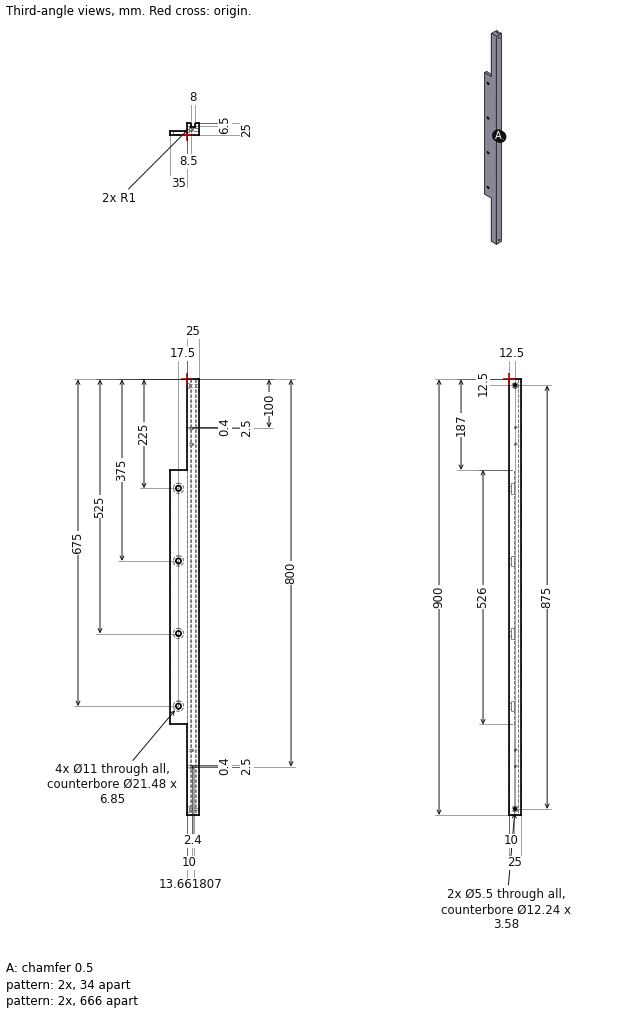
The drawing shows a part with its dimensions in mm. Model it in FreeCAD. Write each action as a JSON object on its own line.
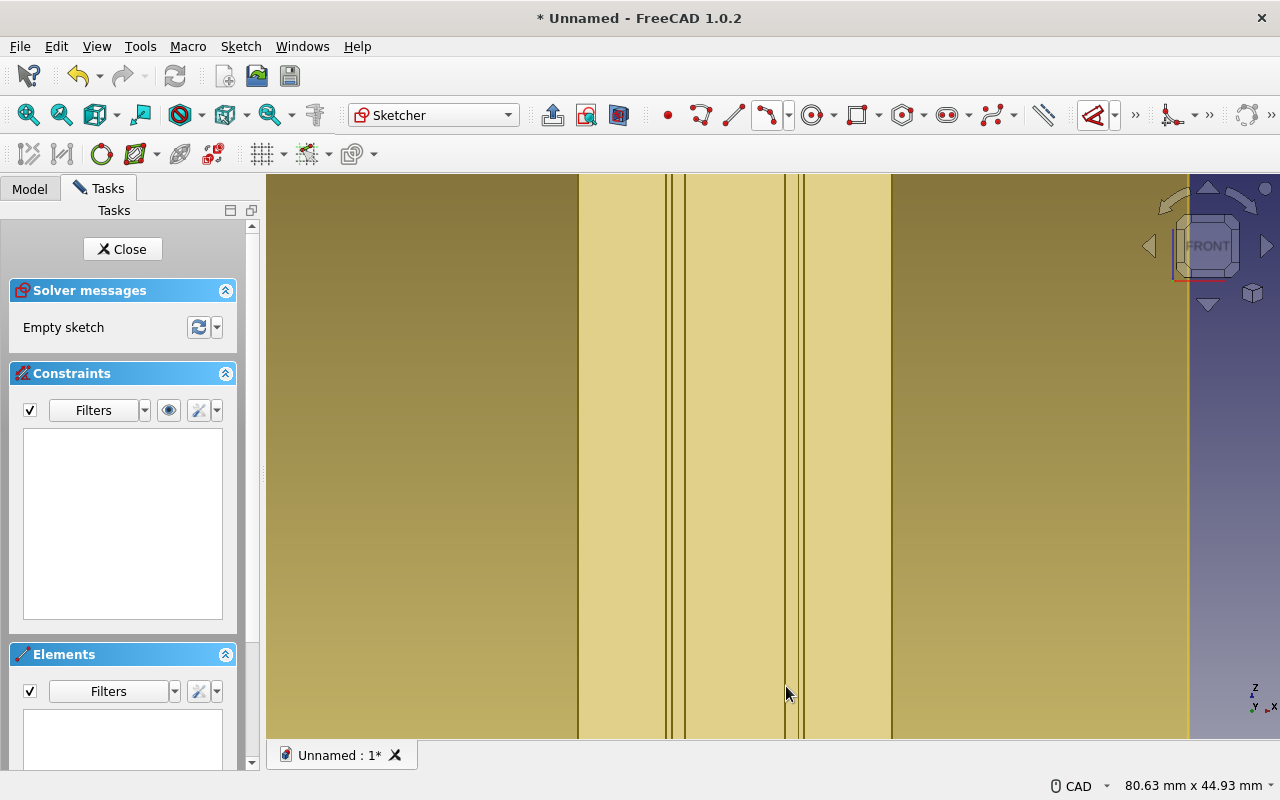
{"action": "scroll", "coordinate": [693, 436], "scroll_direction": "up", "scroll_amount": 4}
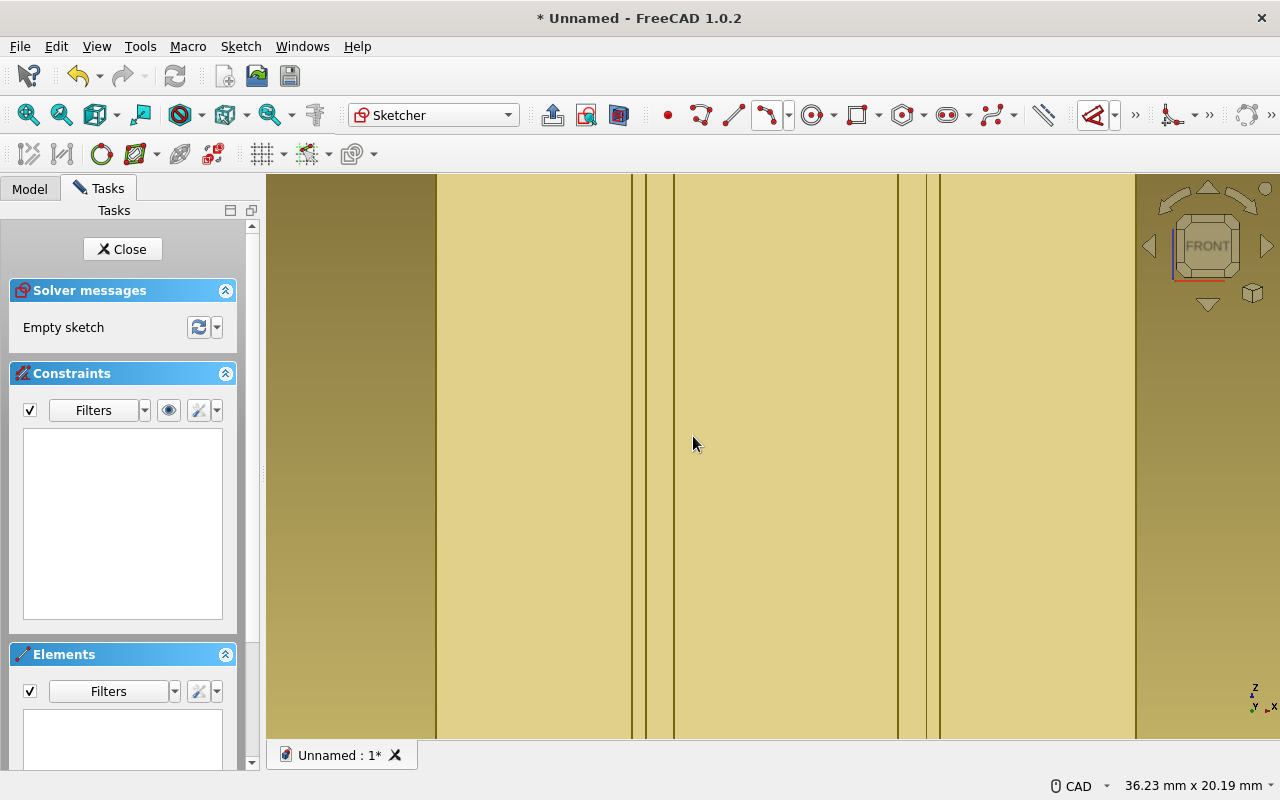
{"action": "left_click", "coordinate": [701, 116]}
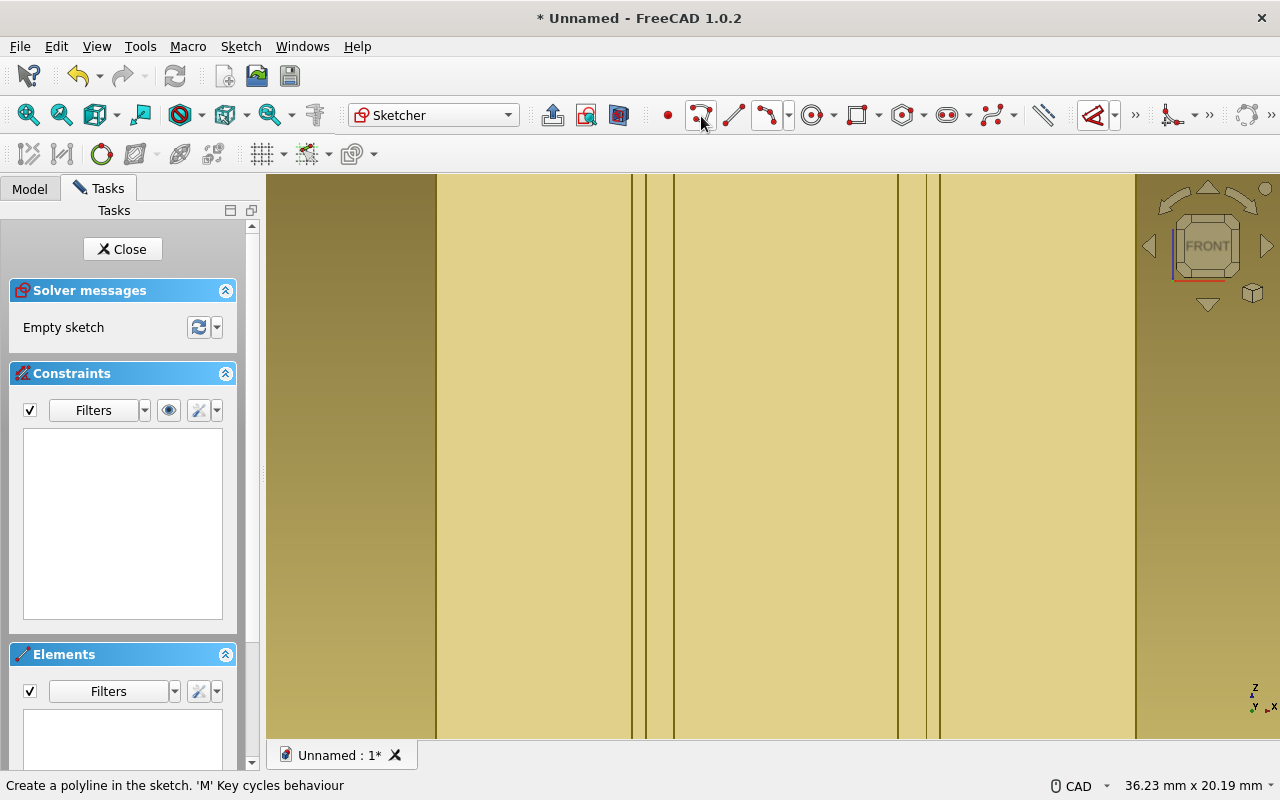
{"action": "left_click", "coordinate": [436, 421]}
{"action": "left_click", "coordinate": [716, 421]}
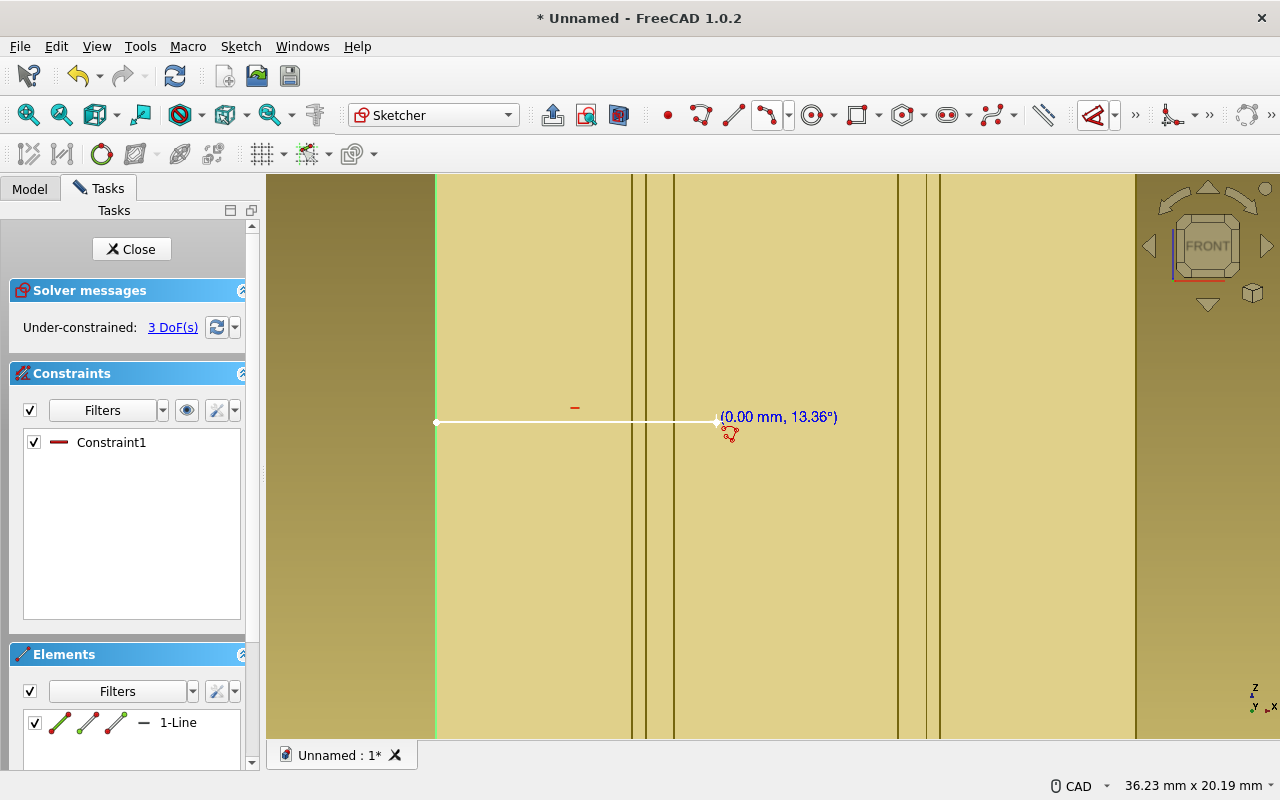
{"action": "scroll", "coordinate": [716, 432], "scroll_direction": "up", "scroll_amount": 2}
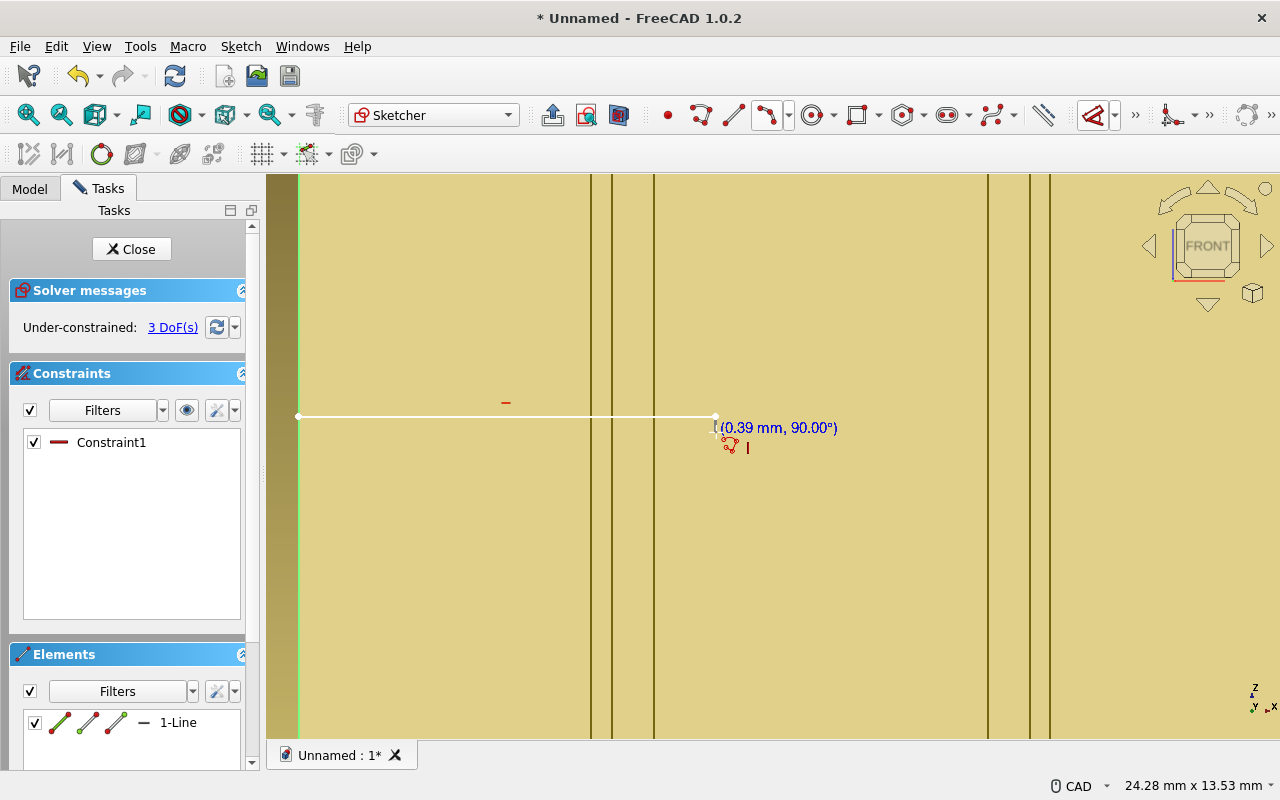
{"action": "left_click", "coordinate": [716, 432]}
{"action": "left_click", "coordinate": [817, 432]}
{"action": "left_click", "coordinate": [869, 519]}
{"action": "left_click", "coordinate": [308, 519]}
{"action": "left_click", "coordinate": [298, 417]}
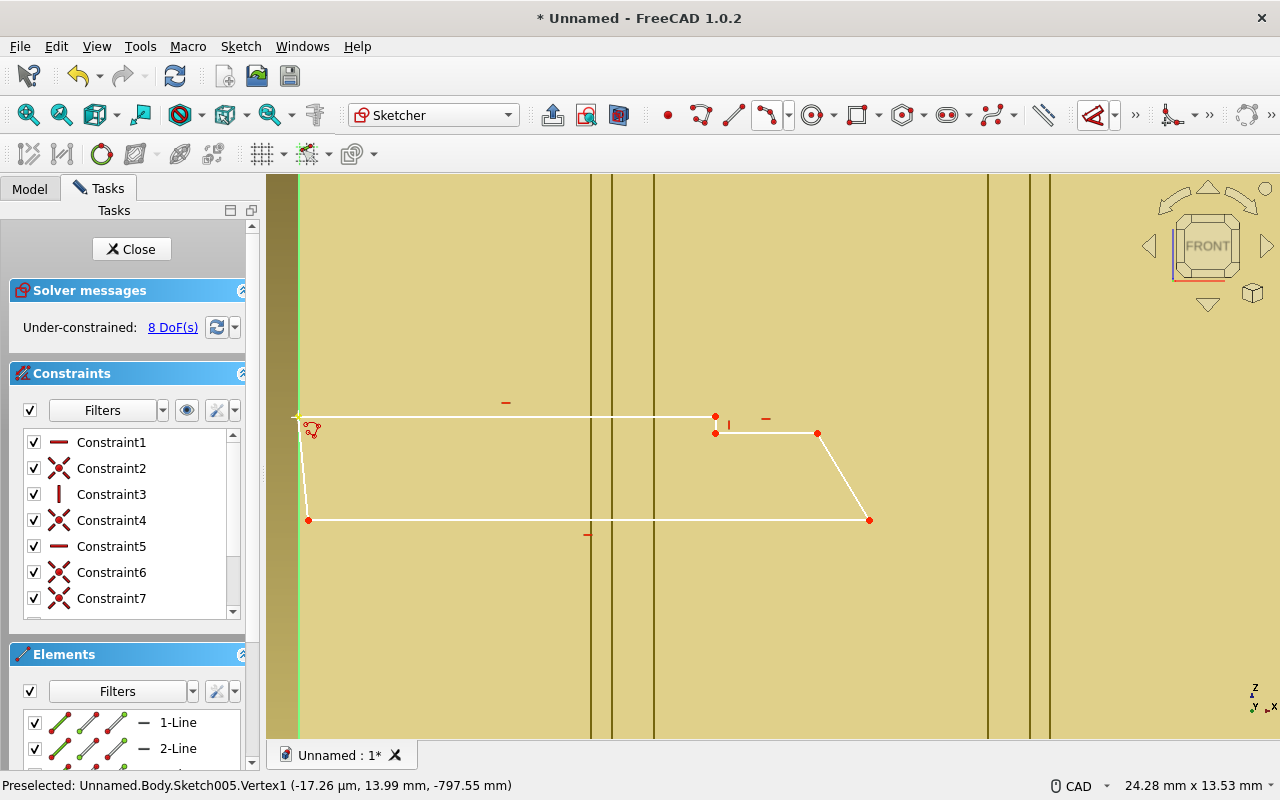
{"action": "left_click", "coordinate": [734, 116]}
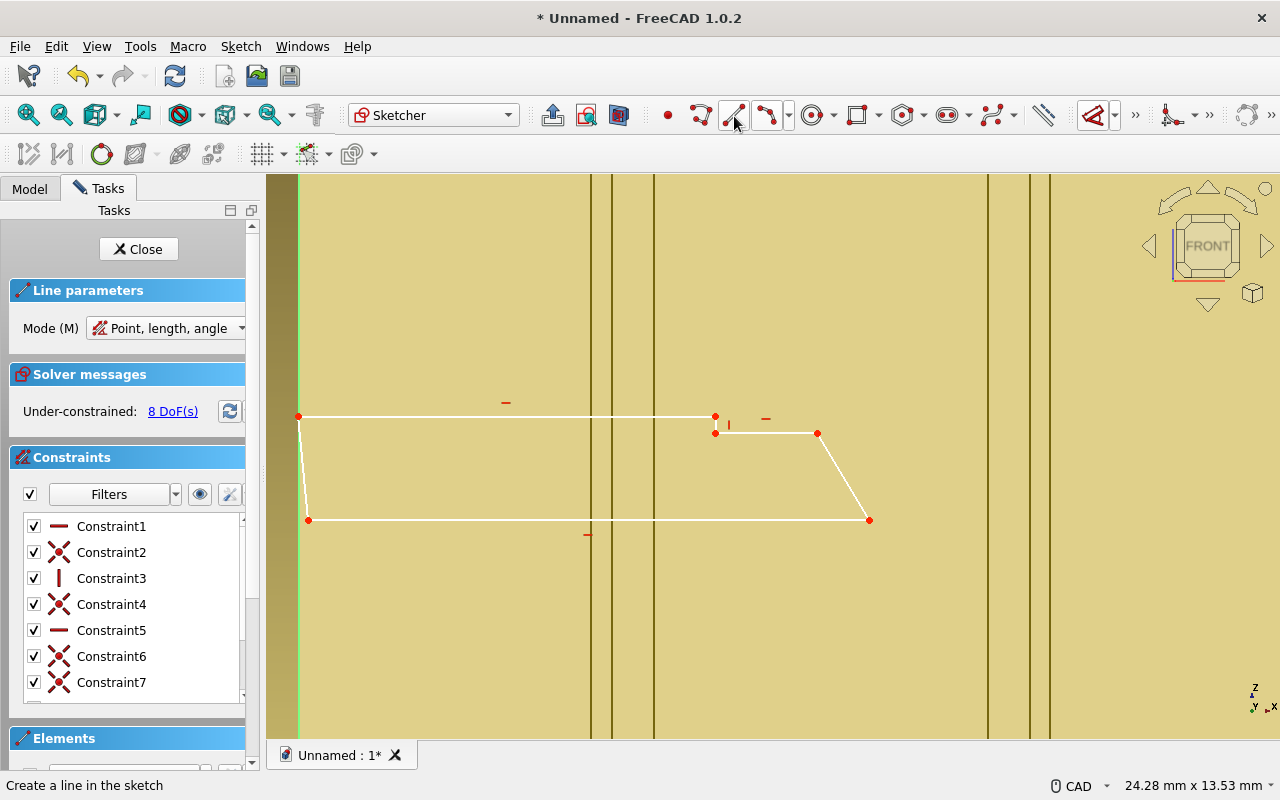
{"action": "left_click", "coordinate": [926, 519]}
{"action": "left_click", "coordinate": [1097, 519]}
{"action": "key", "text": "Escape"}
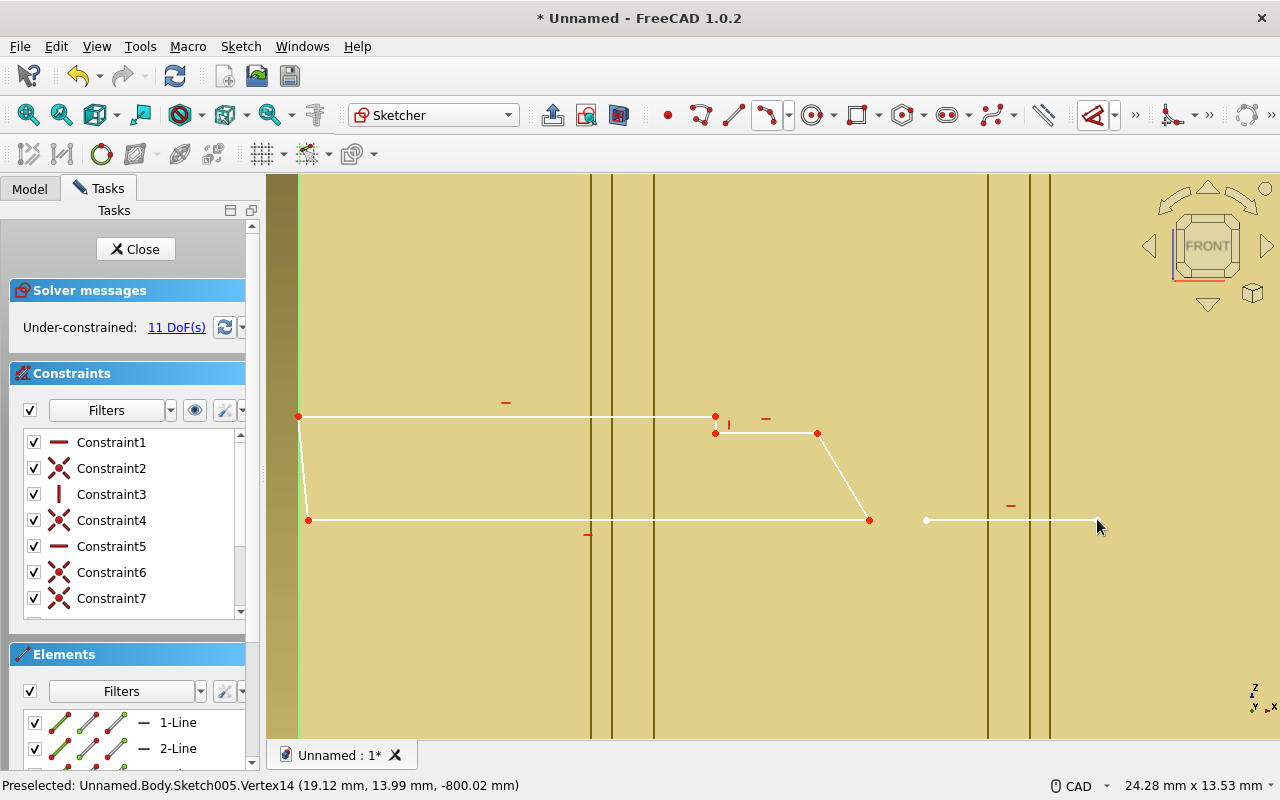
{"action": "left_click", "coordinate": [977, 520]}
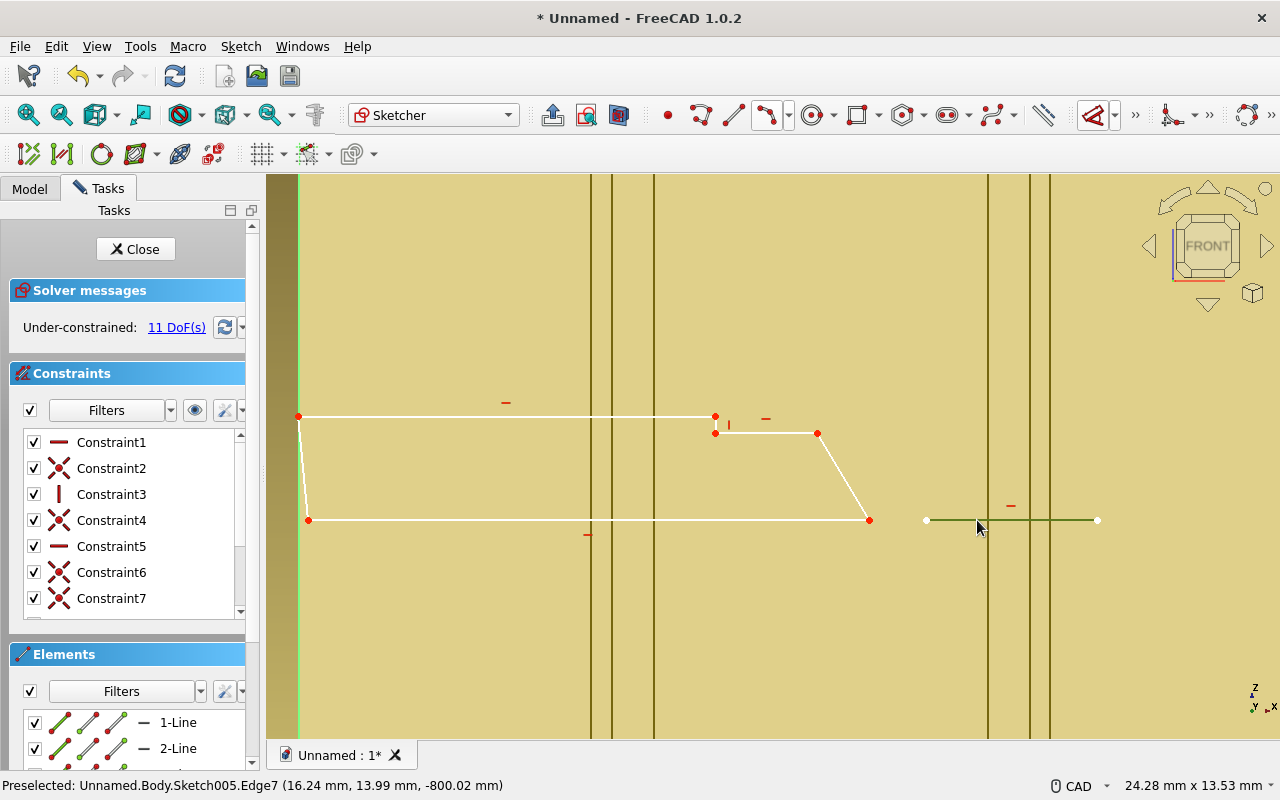
{"action": "left_click", "coordinate": [1044, 116]}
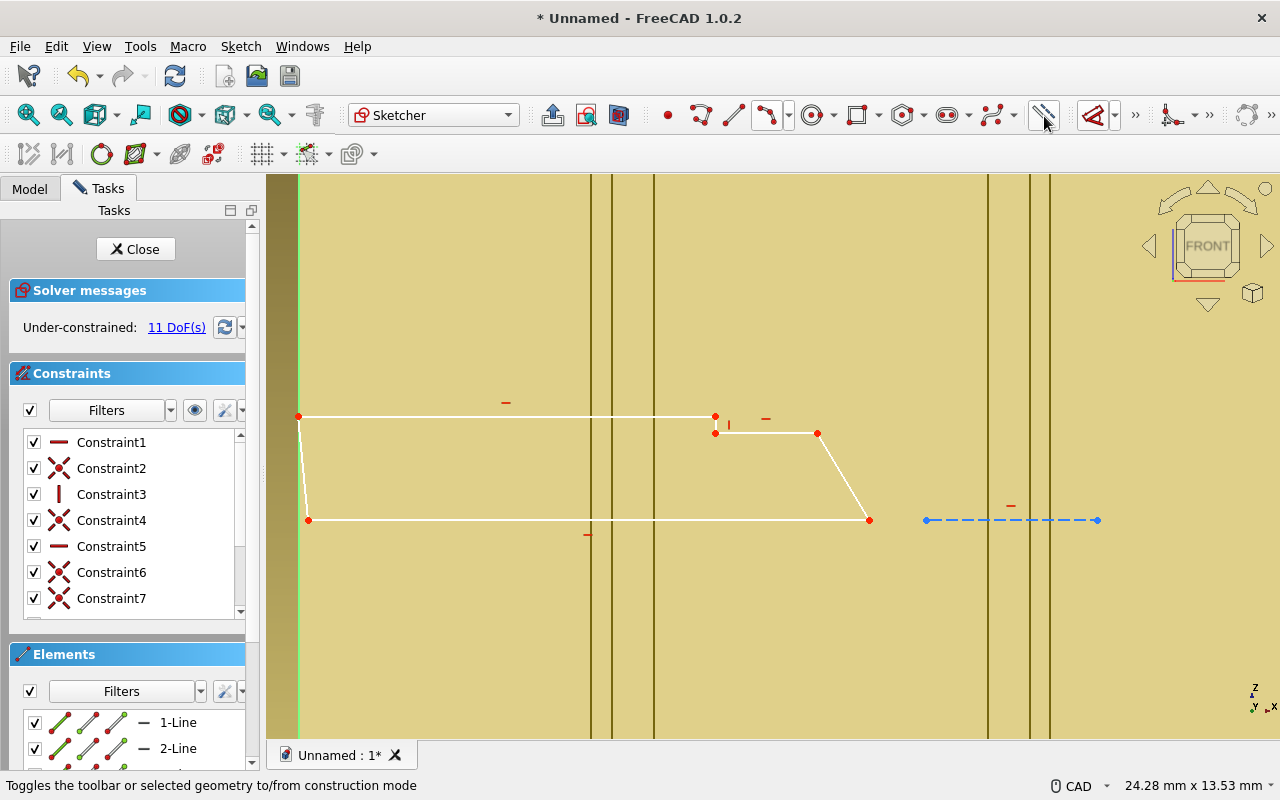
{"action": "left_click", "coordinate": [301, 448]}